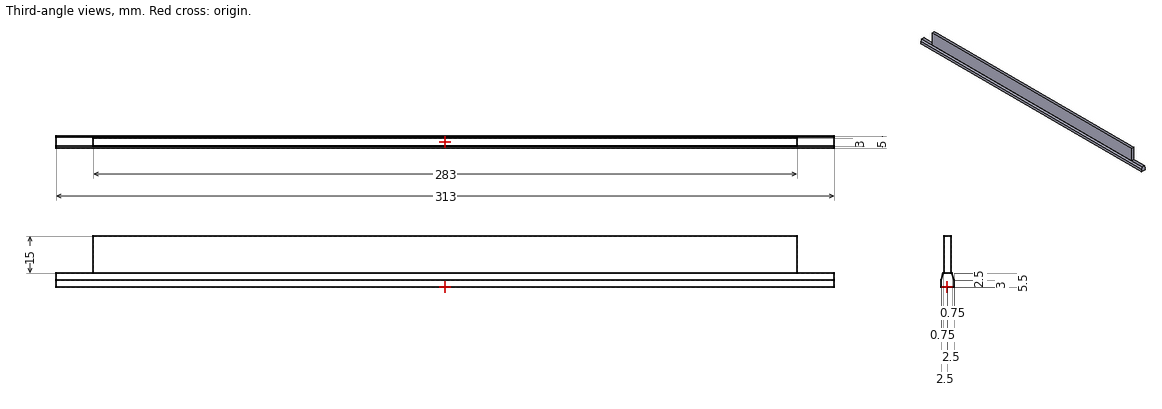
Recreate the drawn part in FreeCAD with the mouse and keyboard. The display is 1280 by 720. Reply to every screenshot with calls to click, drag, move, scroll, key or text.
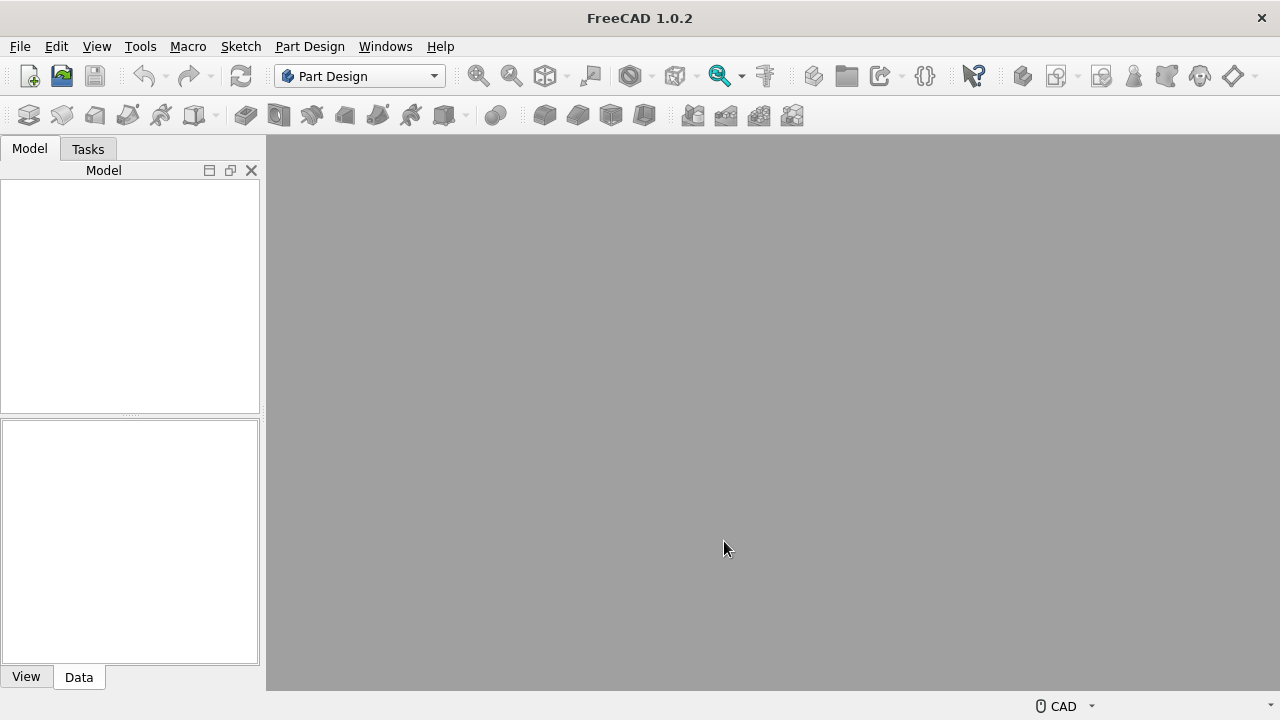
click(29, 76)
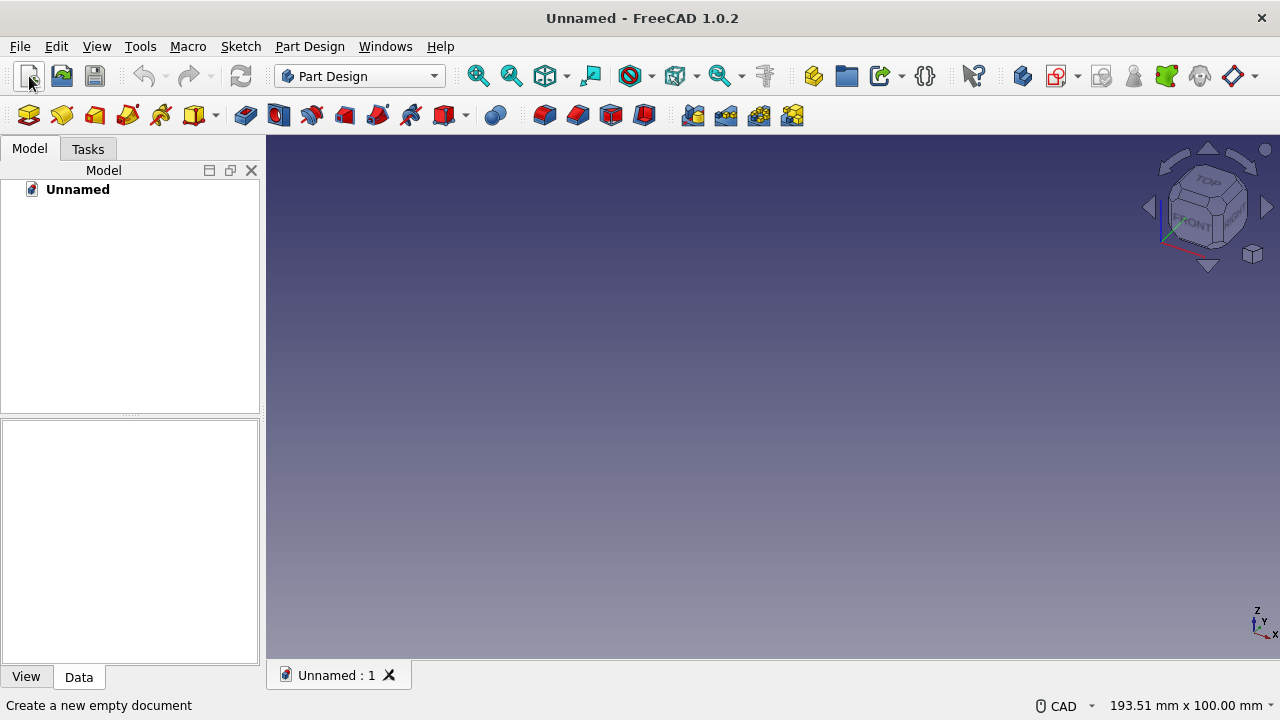
click(1056, 76)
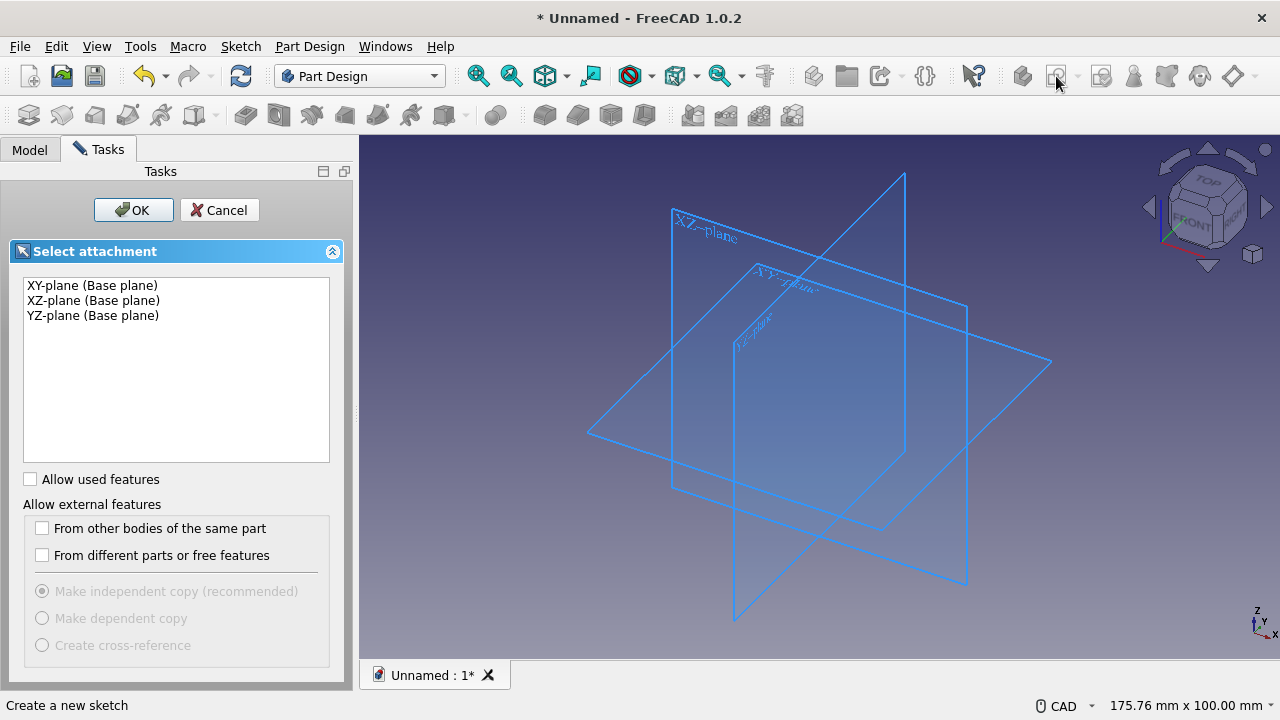
click(84, 286)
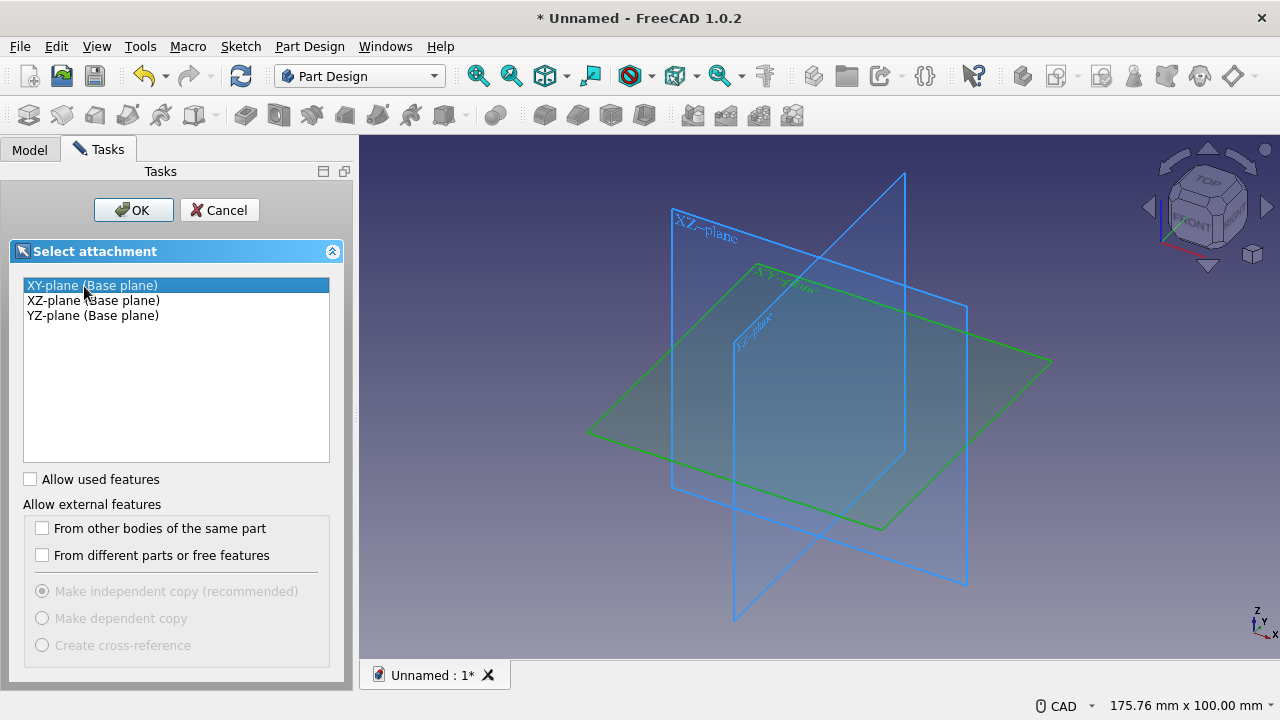
click(134, 210)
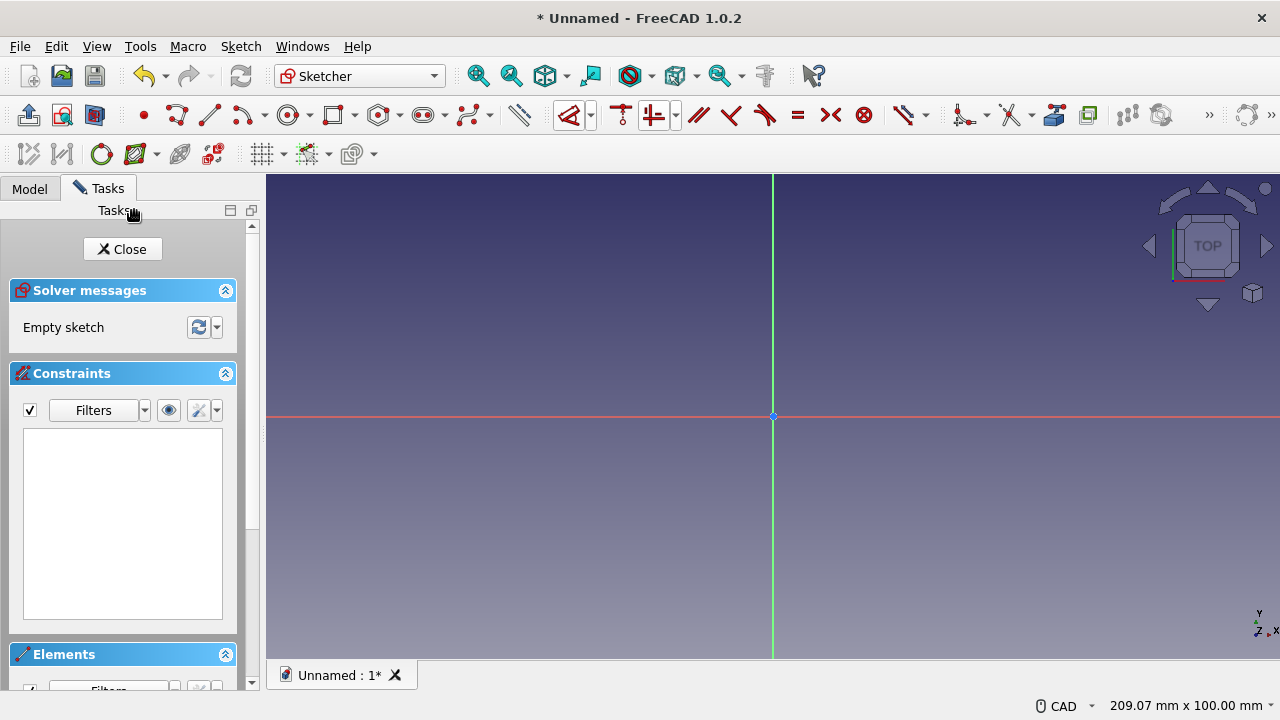
scroll(665, 417, down, 5)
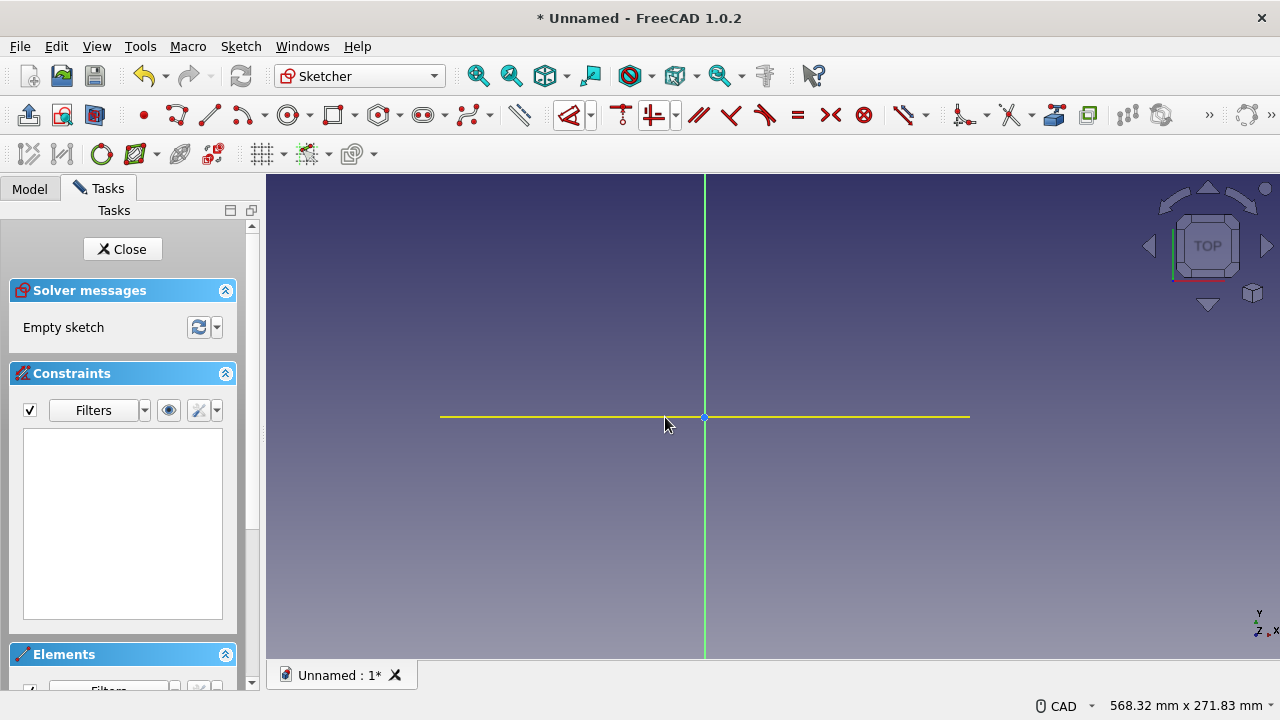
key(g)
key(v)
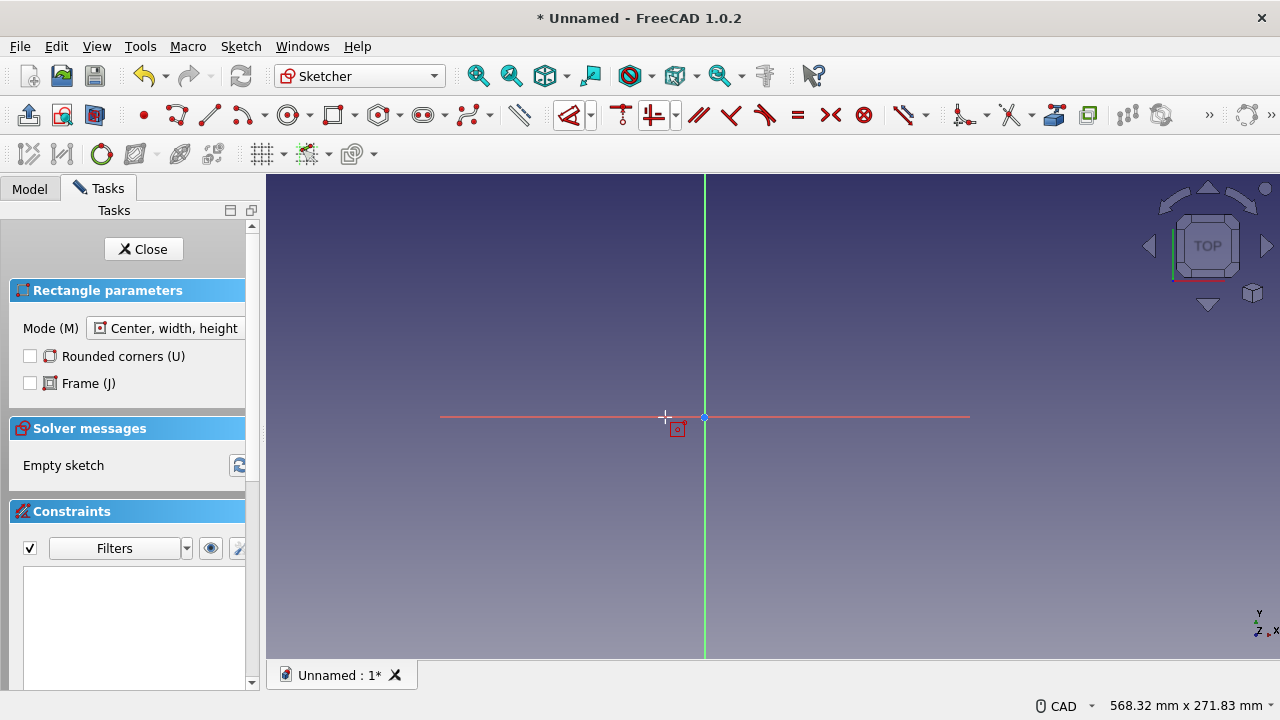
scroll(705, 417, up, 7)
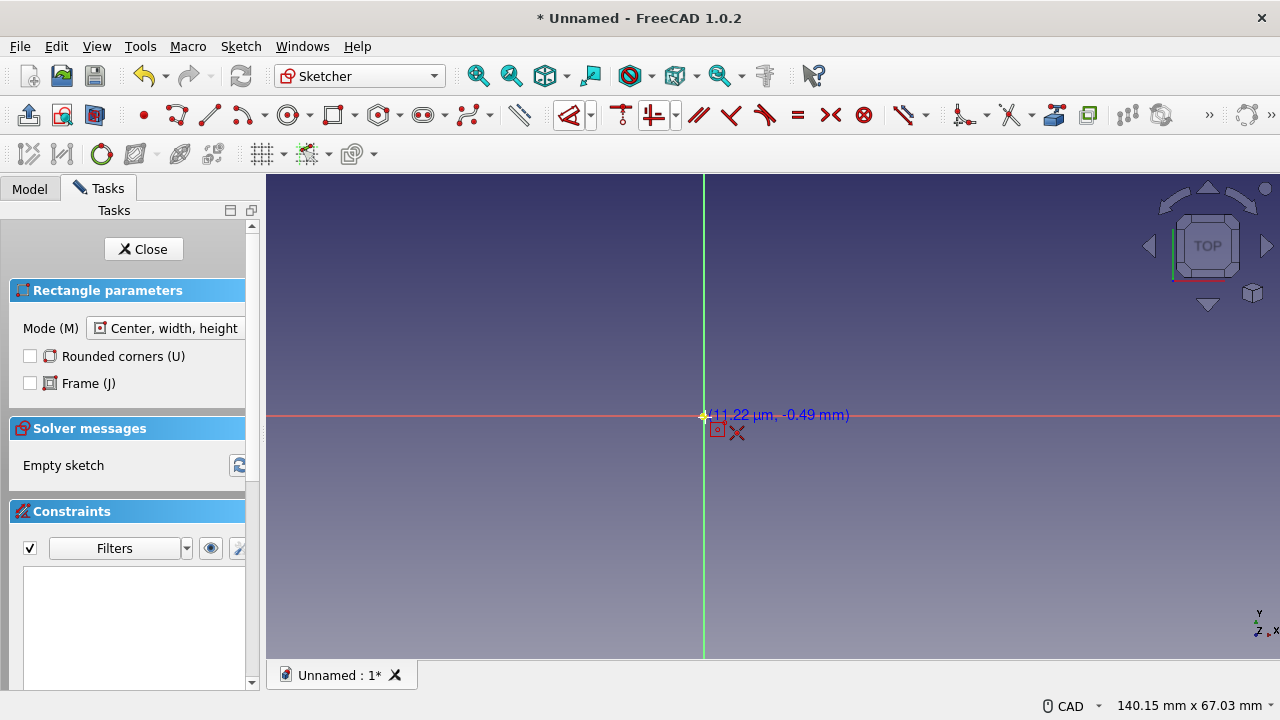
scroll(705, 417, down, 7)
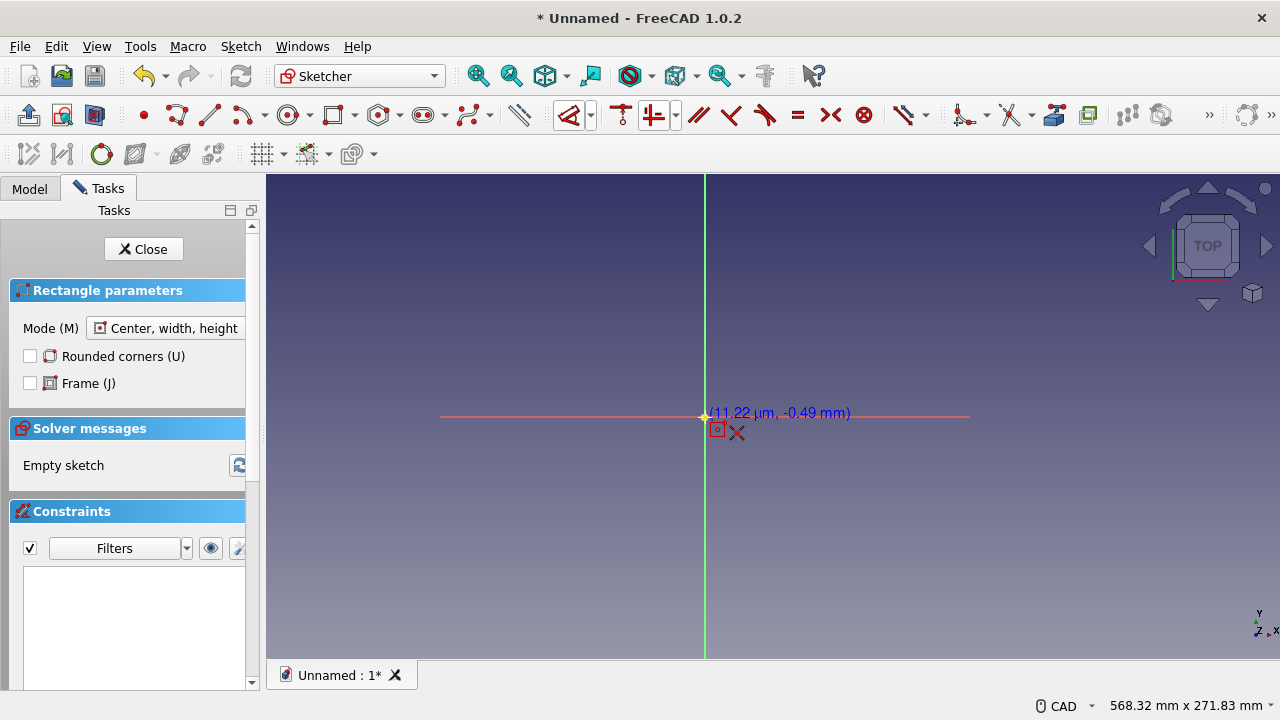
click(705, 417)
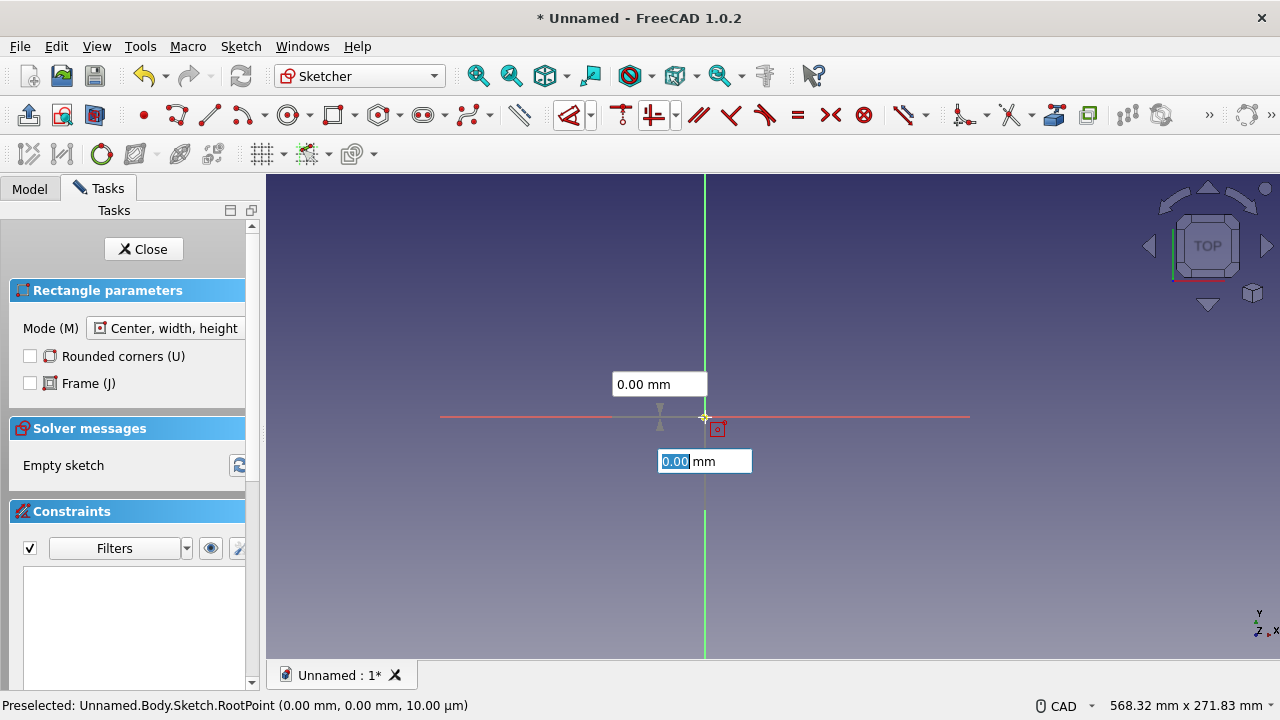
scroll(984, 413, up, 7)
move(983, 410)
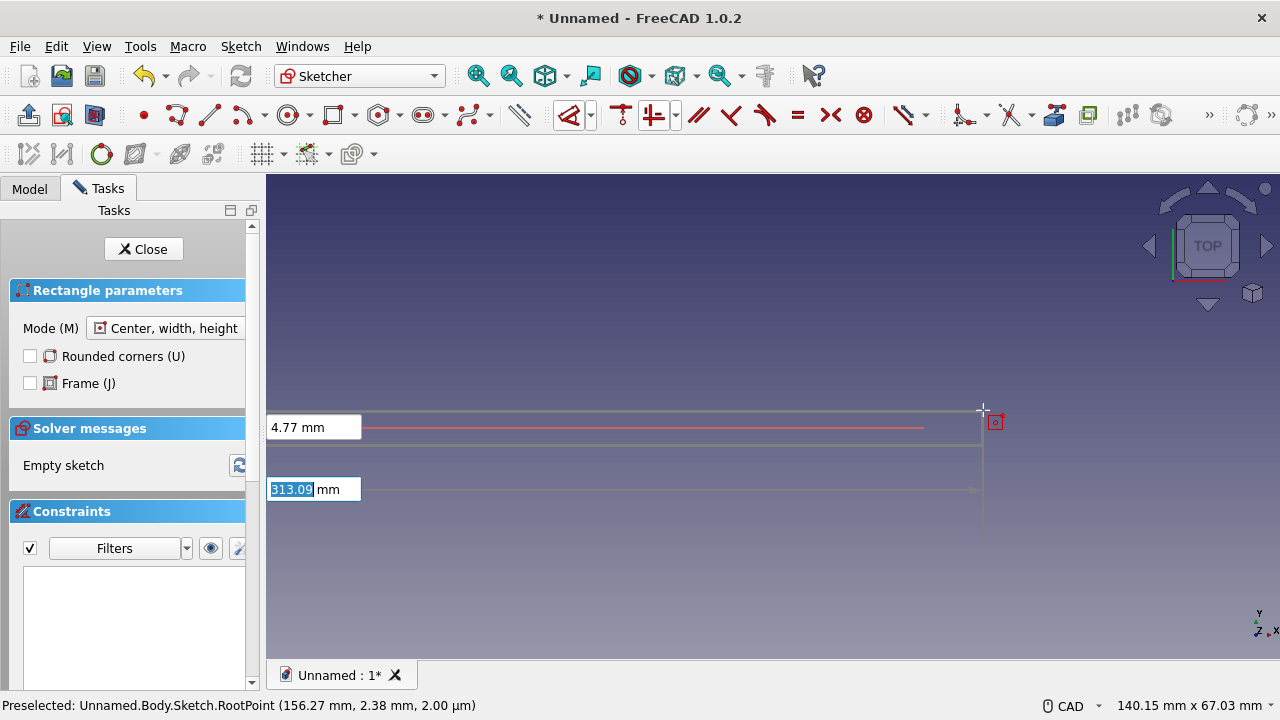
text(313)
key(Tab)
text(5)
key(Return)
key(Escape)